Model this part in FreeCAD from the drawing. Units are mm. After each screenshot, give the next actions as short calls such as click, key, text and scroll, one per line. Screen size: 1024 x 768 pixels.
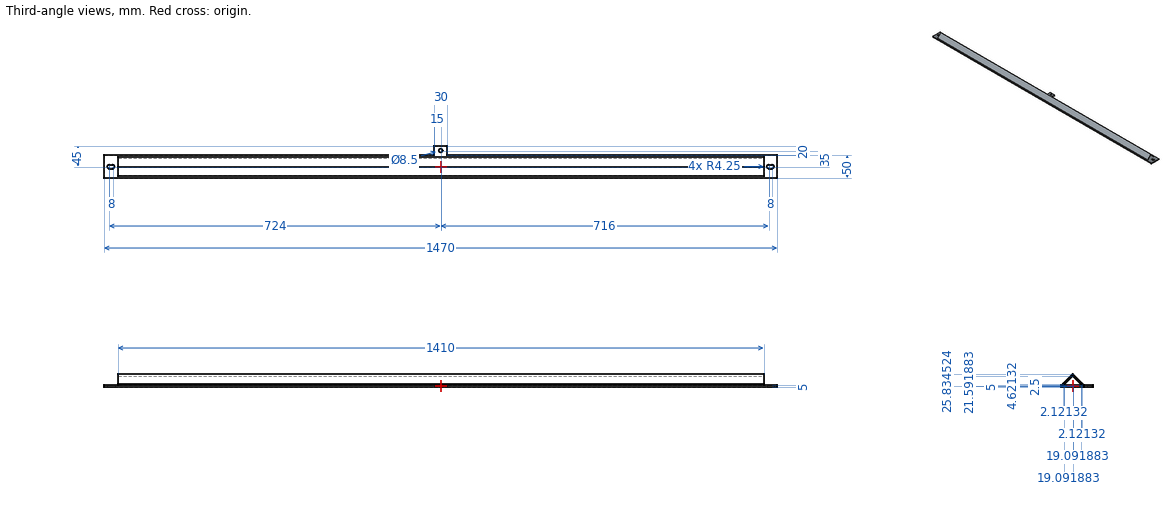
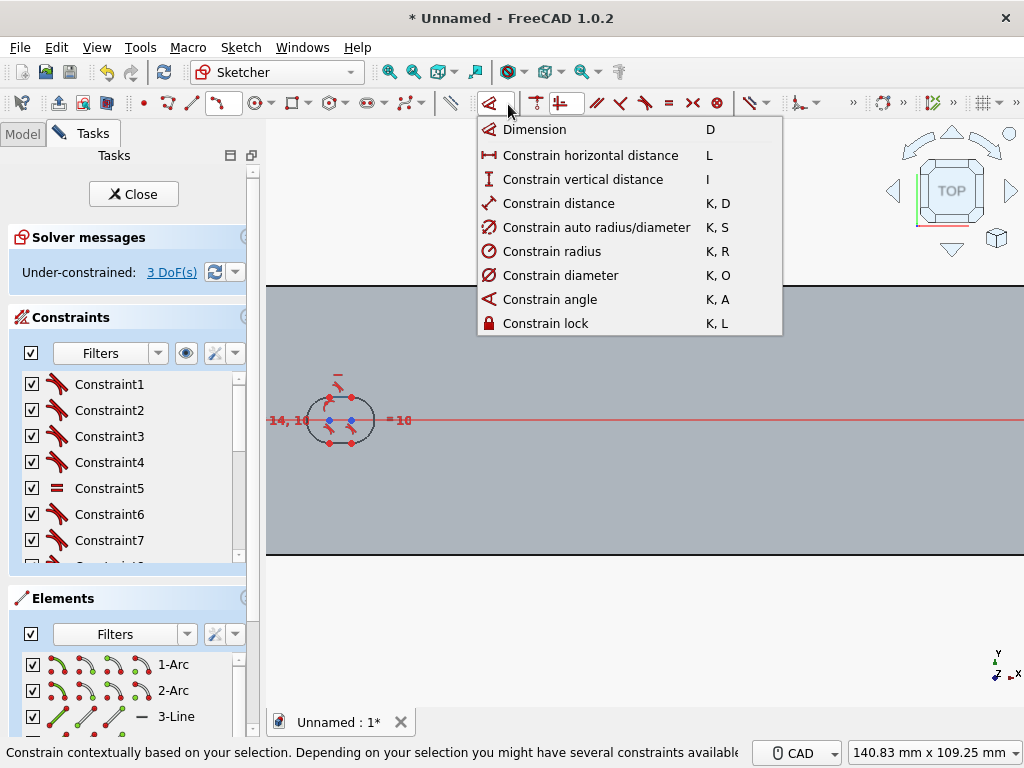
click(630, 155)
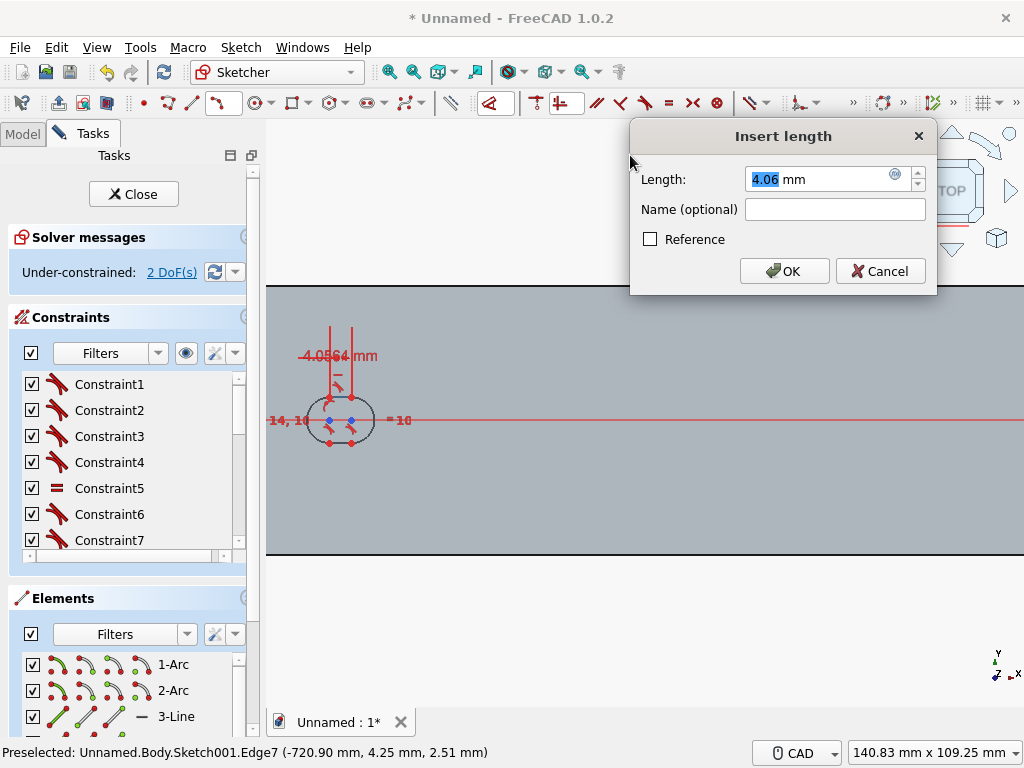
text(8)
key(Return)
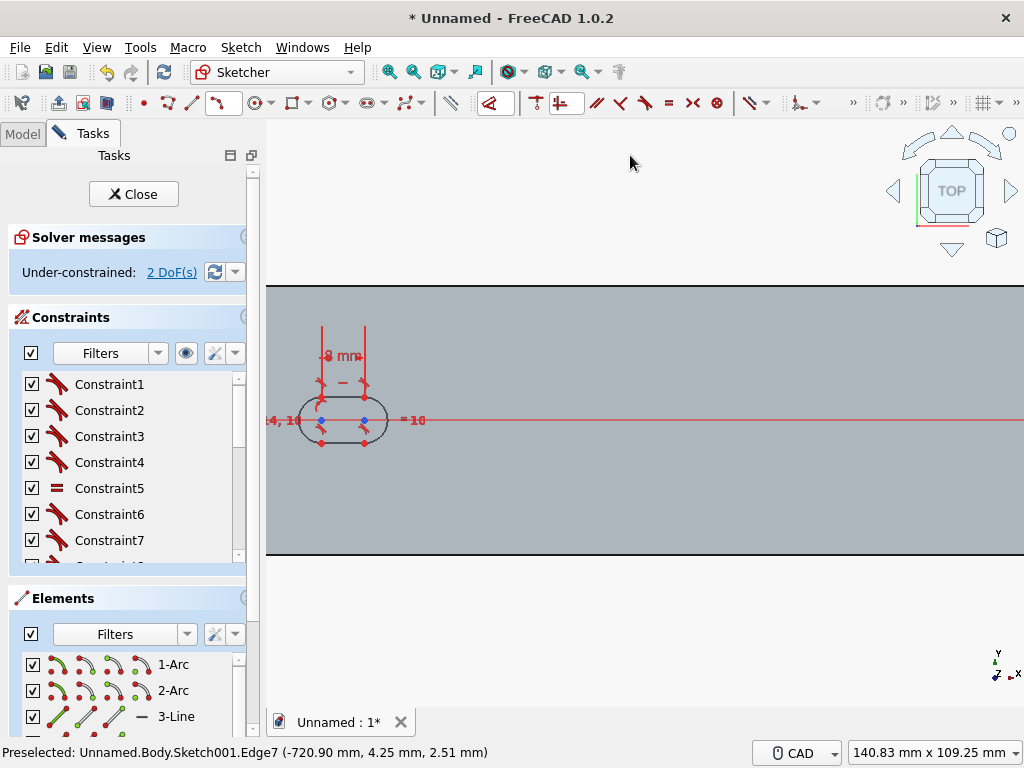
scroll(386, 413, down, 15)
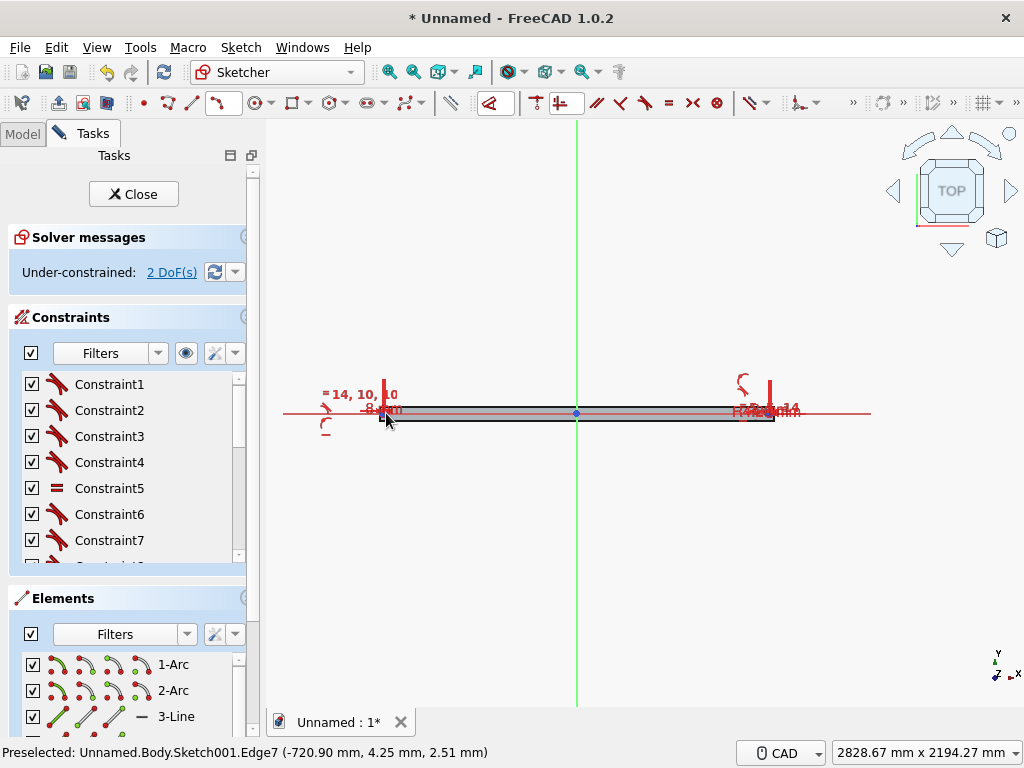
scroll(769, 413, up, 12)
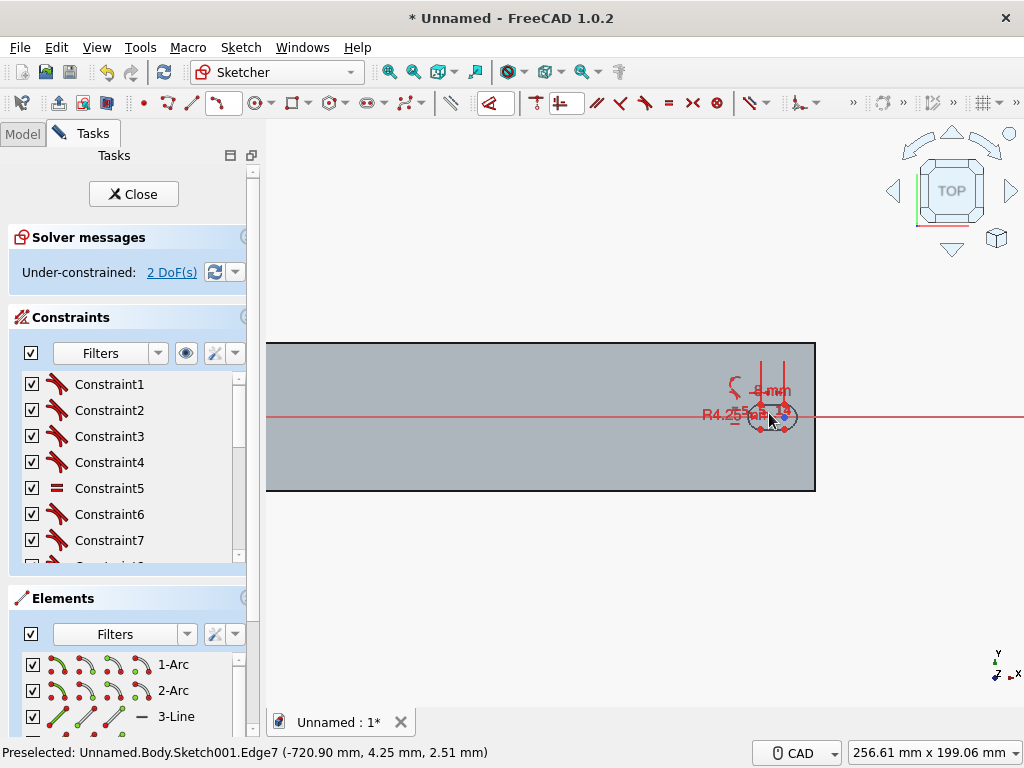
click(761, 405)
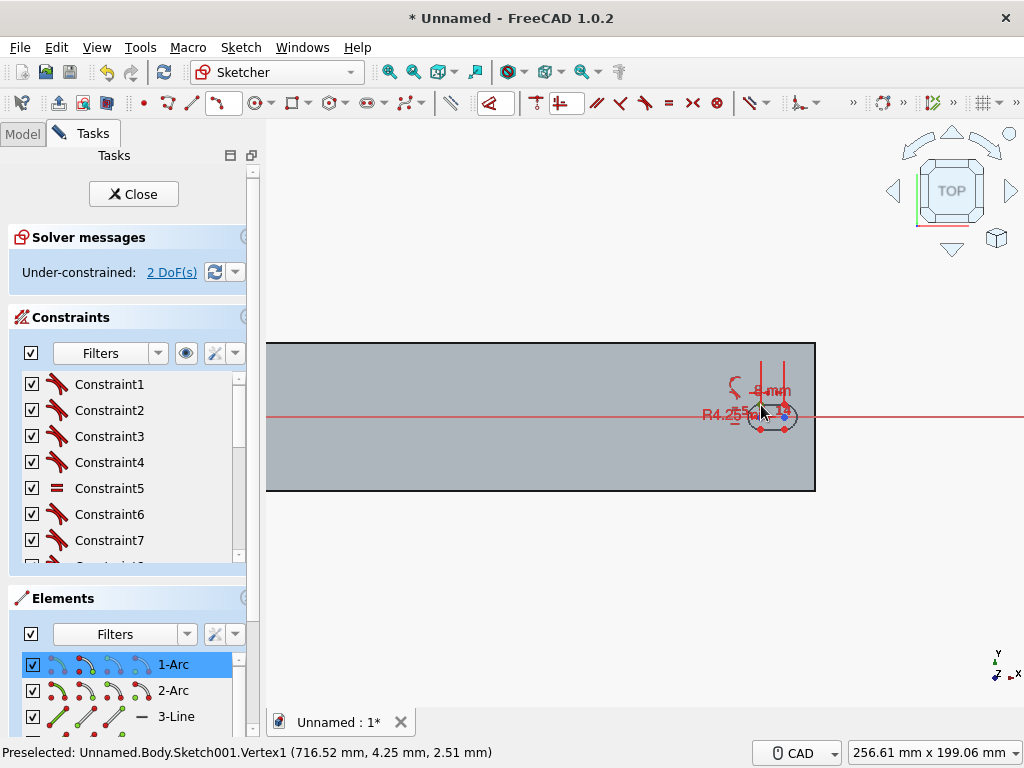
click(508, 104)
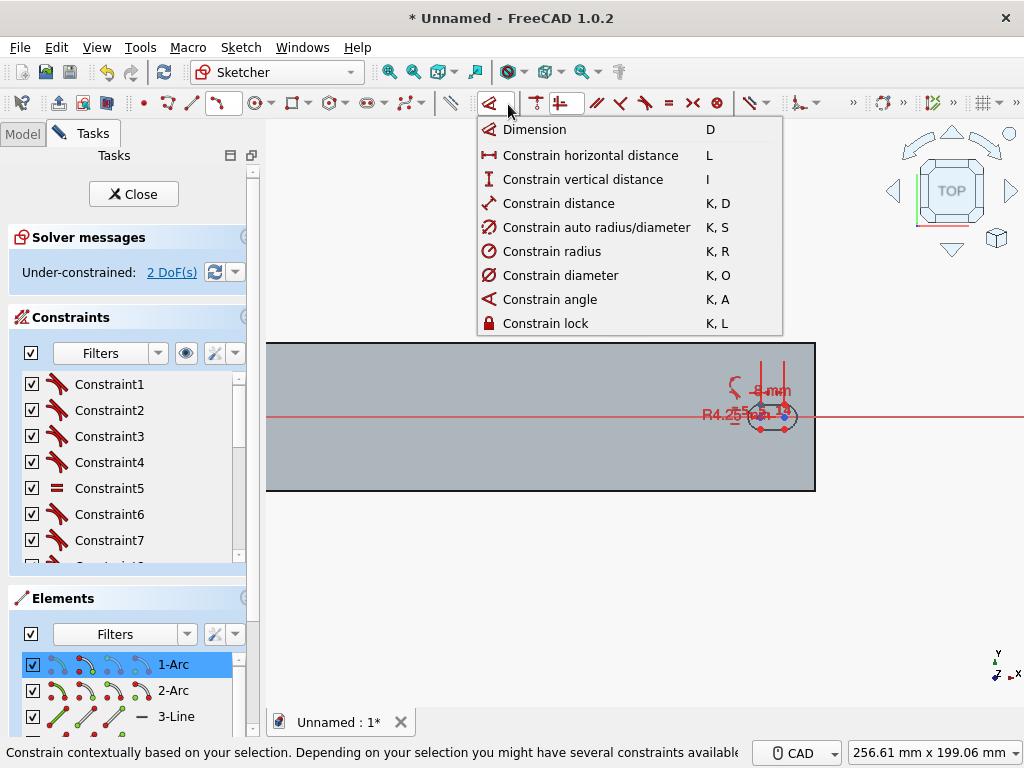
click(630, 155)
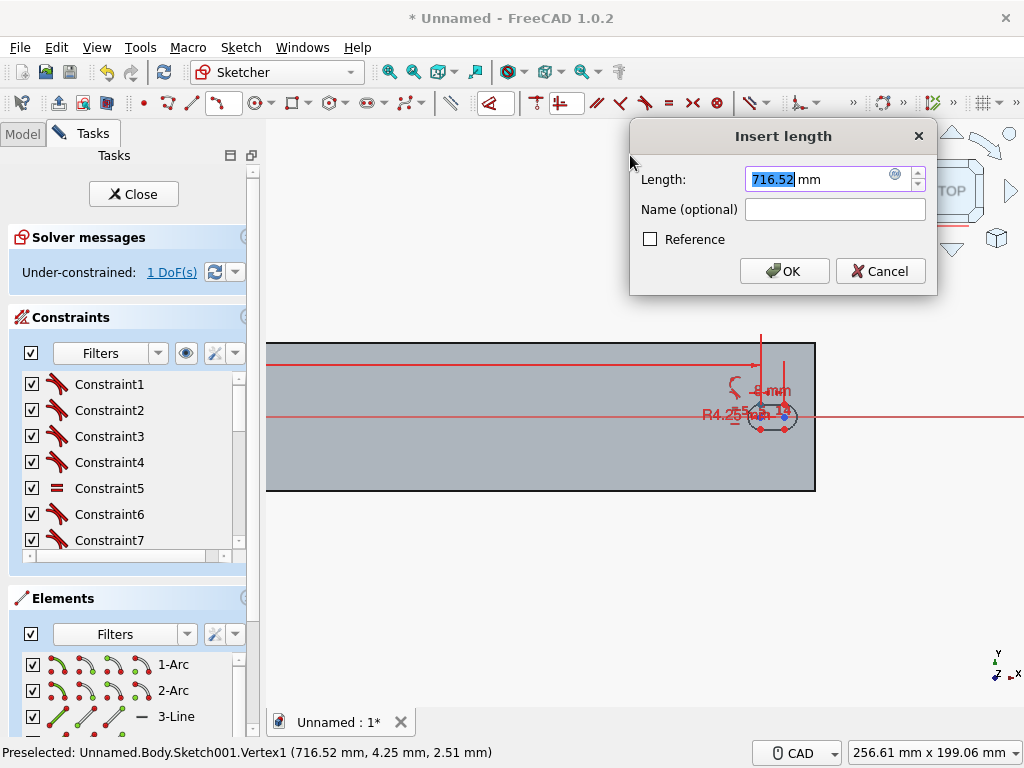
text(716)
key(Return)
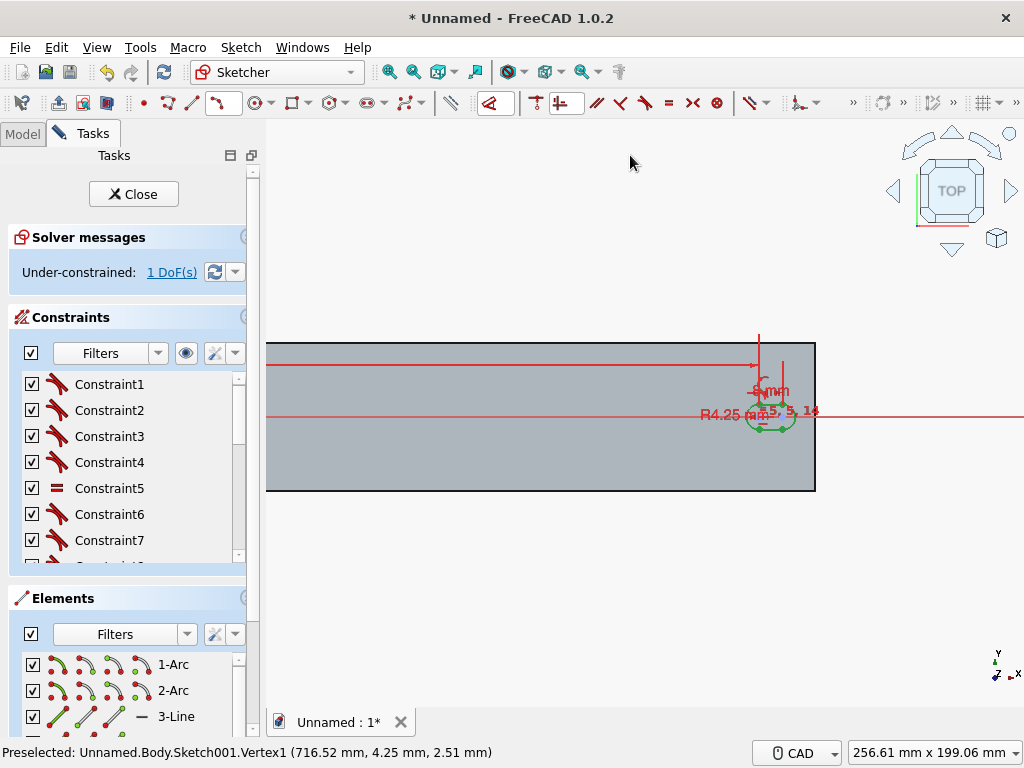
scroll(769, 413, down, 12)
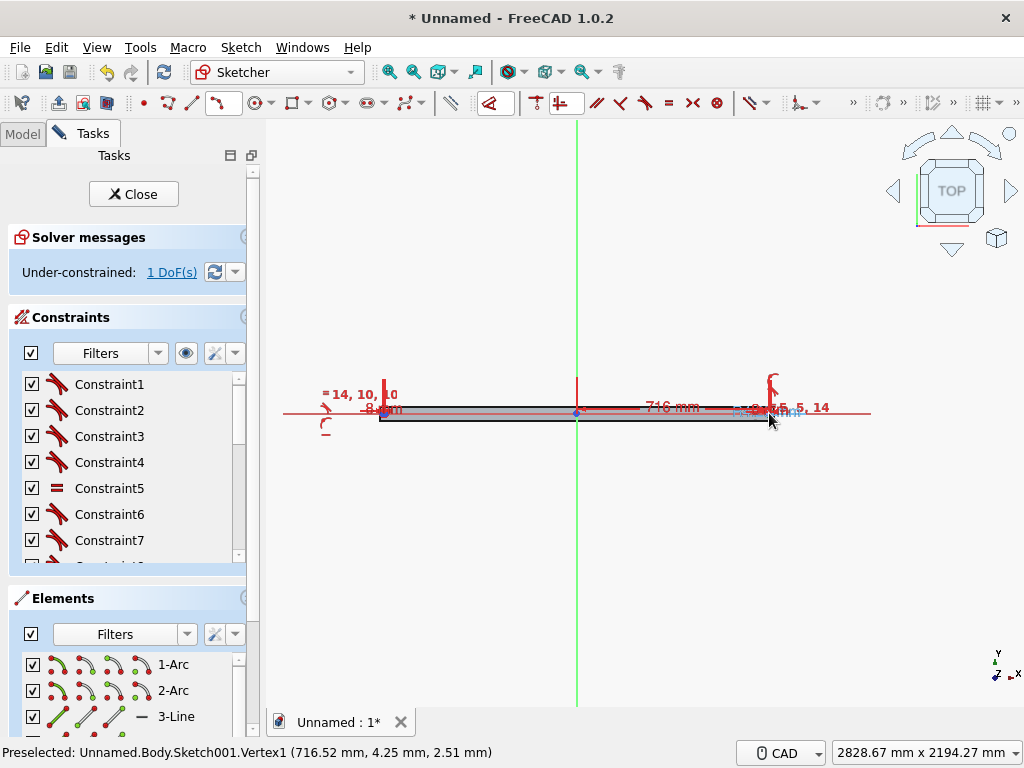
scroll(383, 413, up, 12)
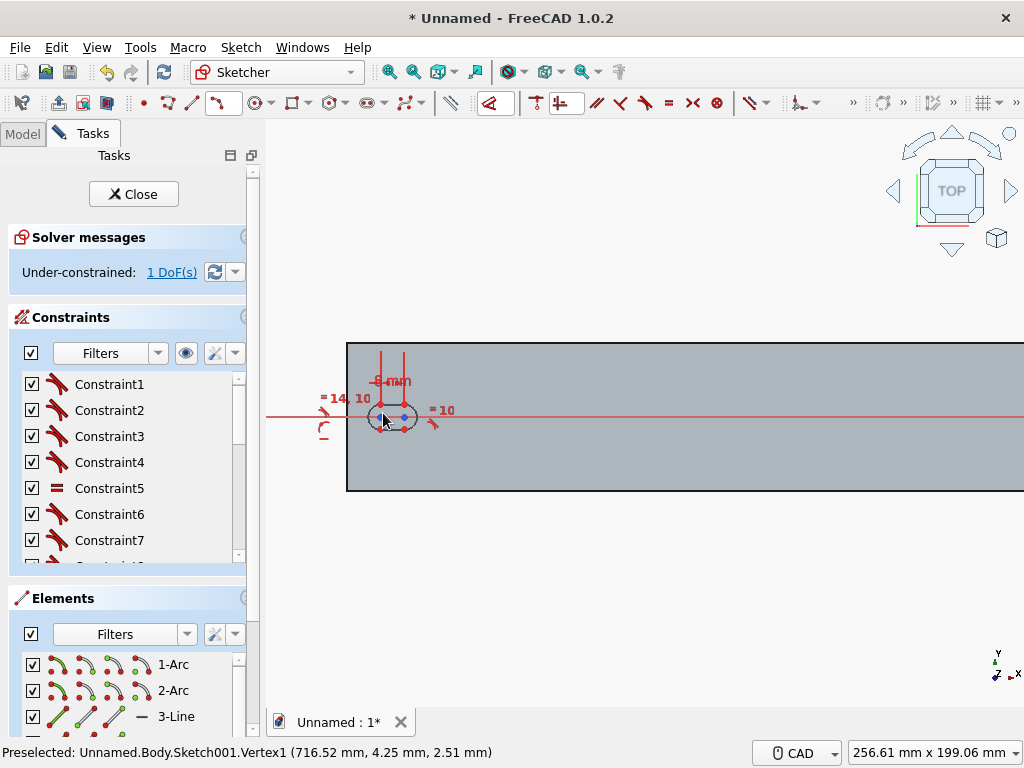
click(381, 405)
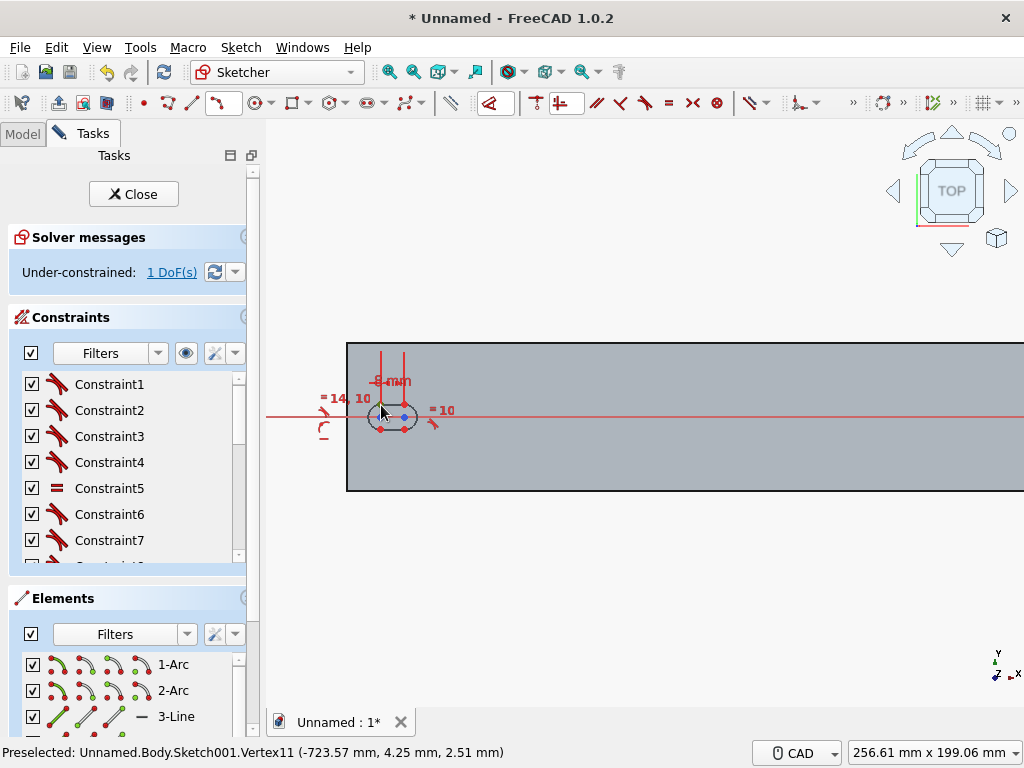
click(508, 104)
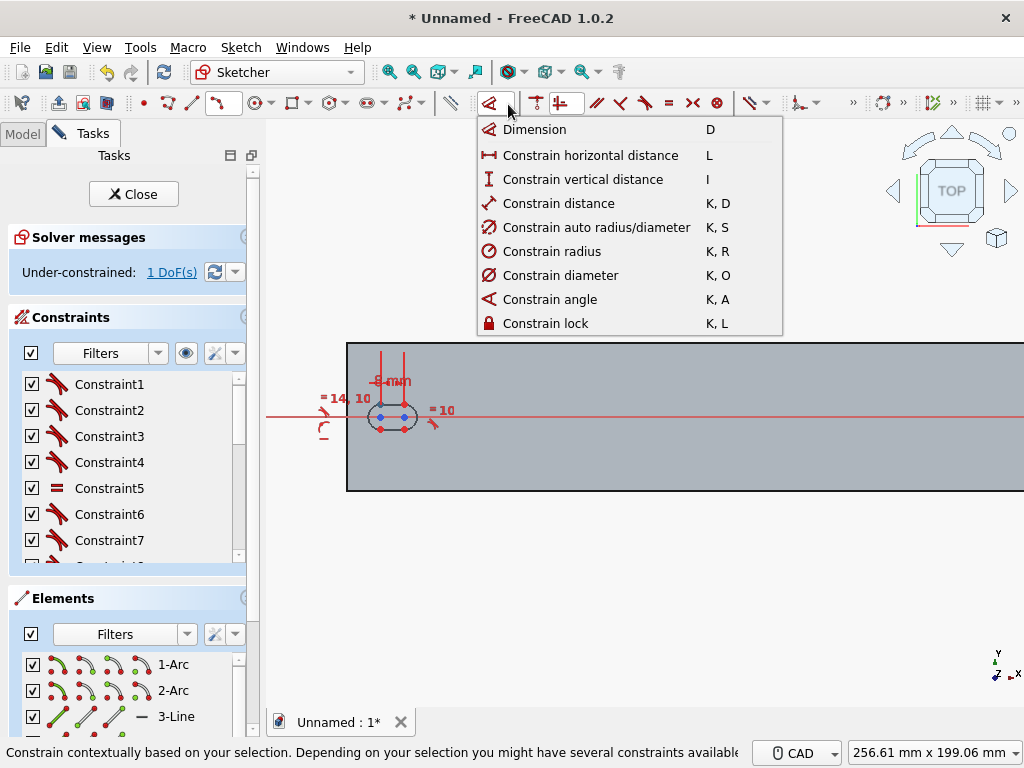
click(630, 155)